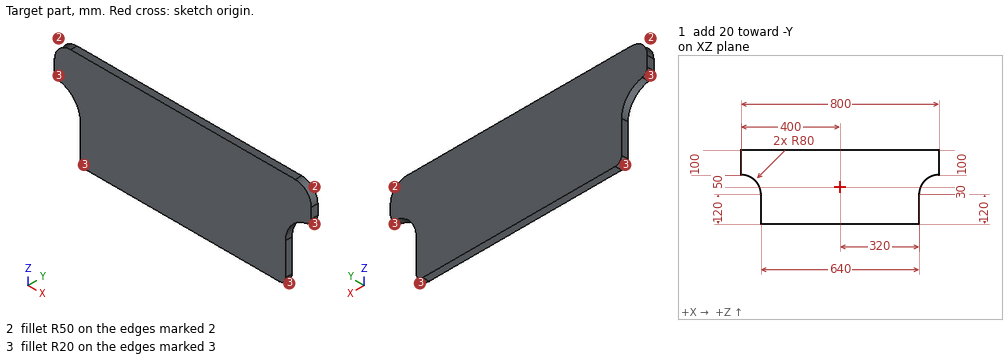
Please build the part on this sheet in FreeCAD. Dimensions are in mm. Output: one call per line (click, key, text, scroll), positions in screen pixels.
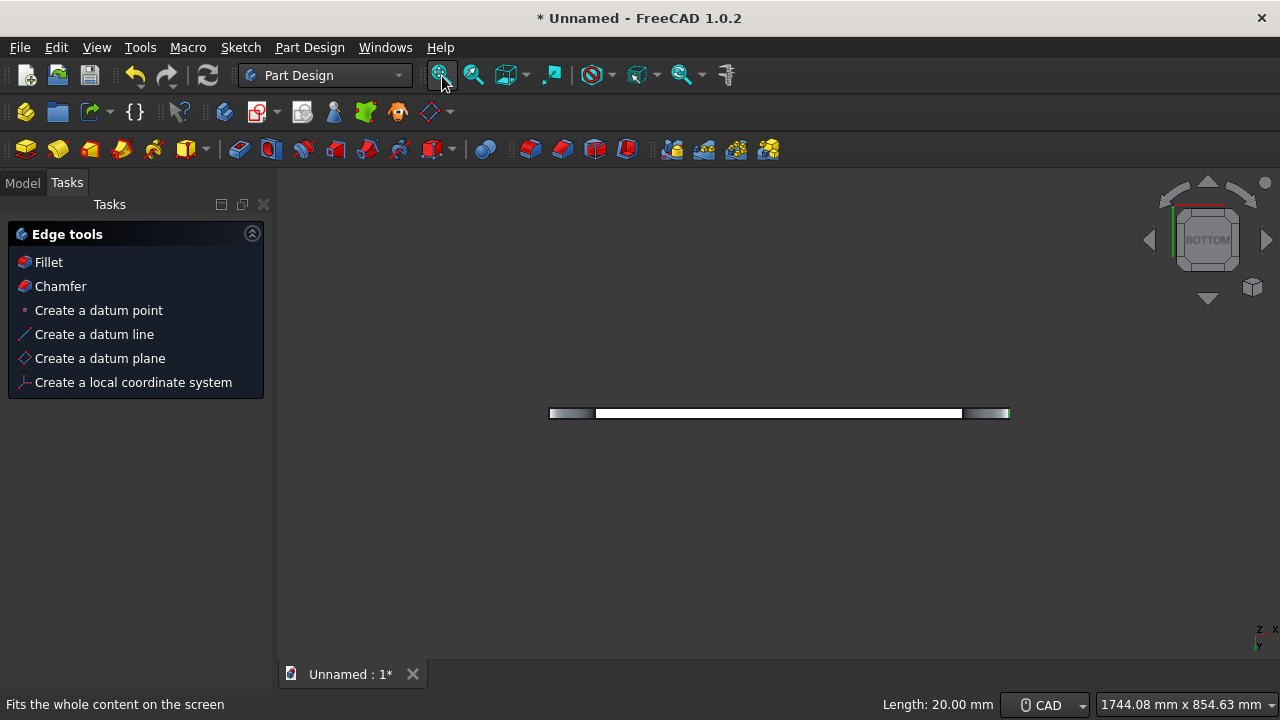
click(595, 414, ctrl)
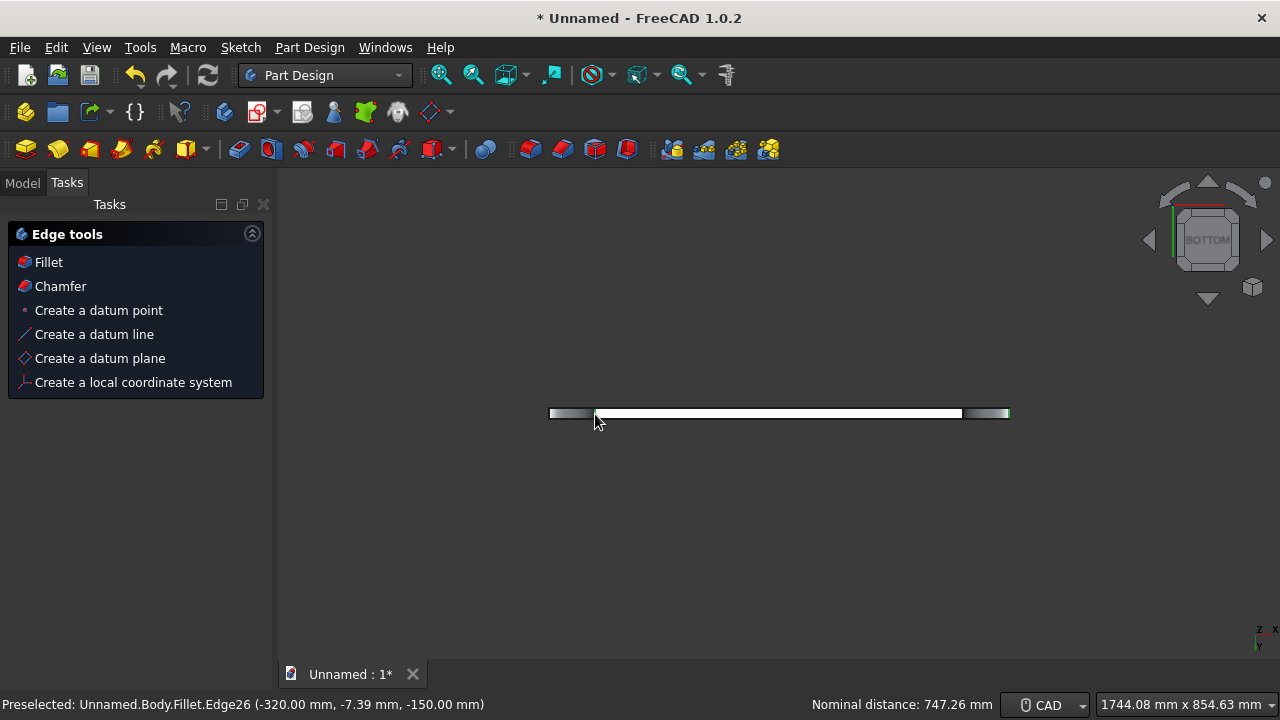
click(963, 414, ctrl)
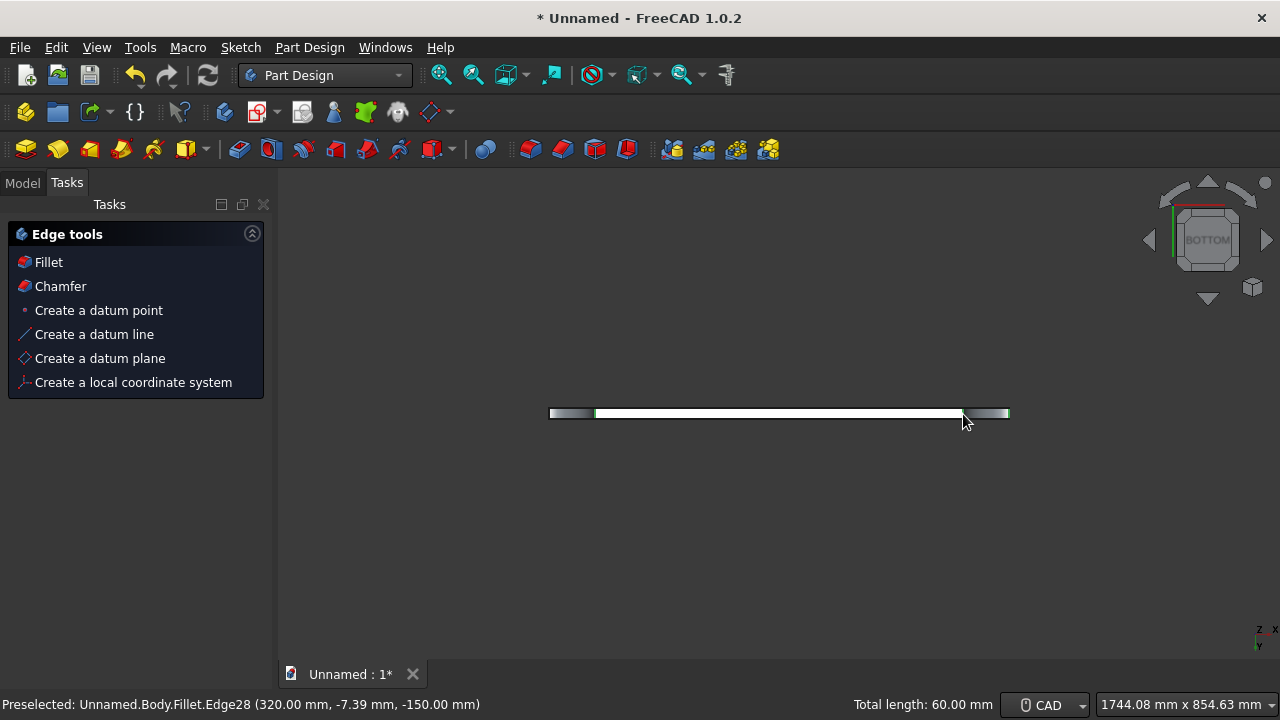
scroll(549, 412, up, 7)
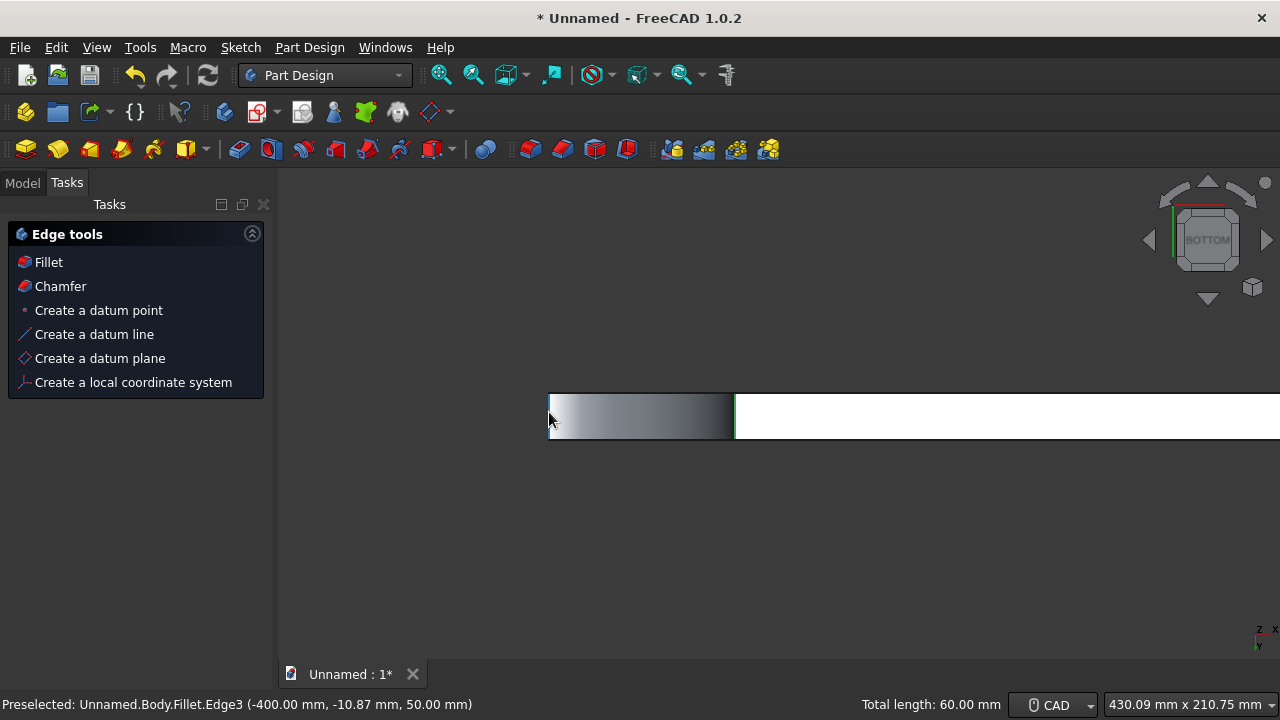
click(442, 76)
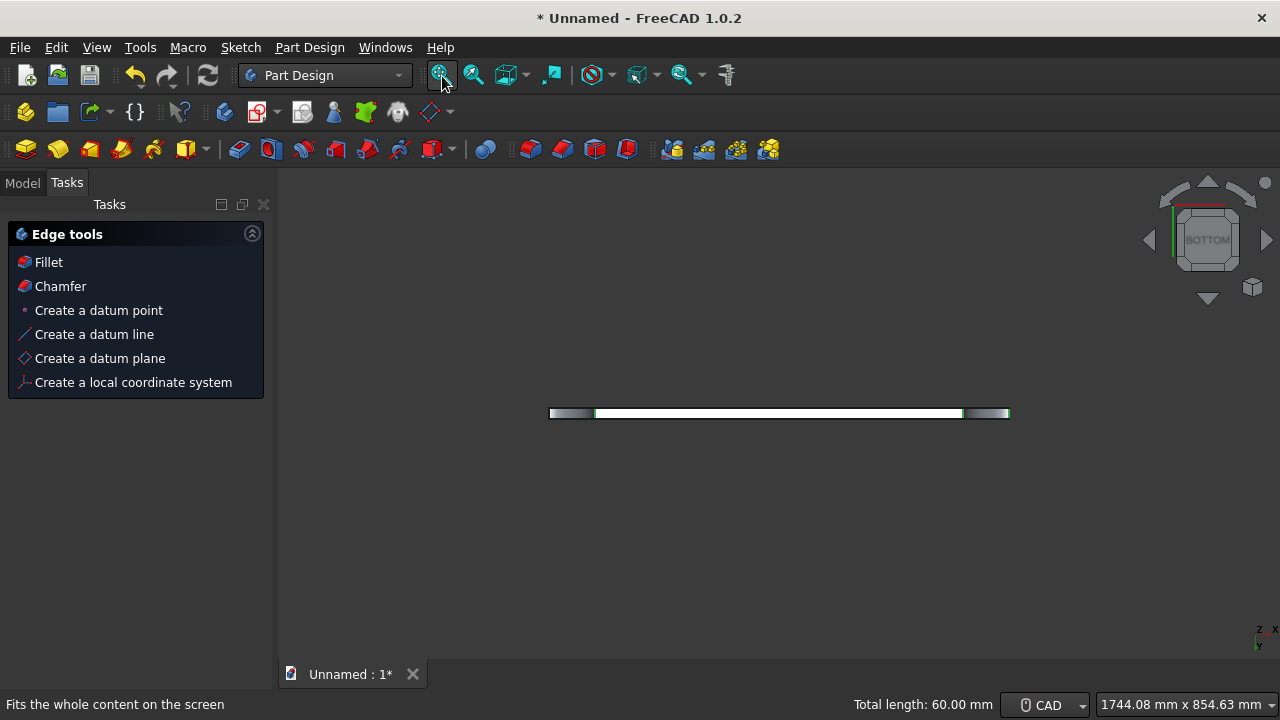
key(4)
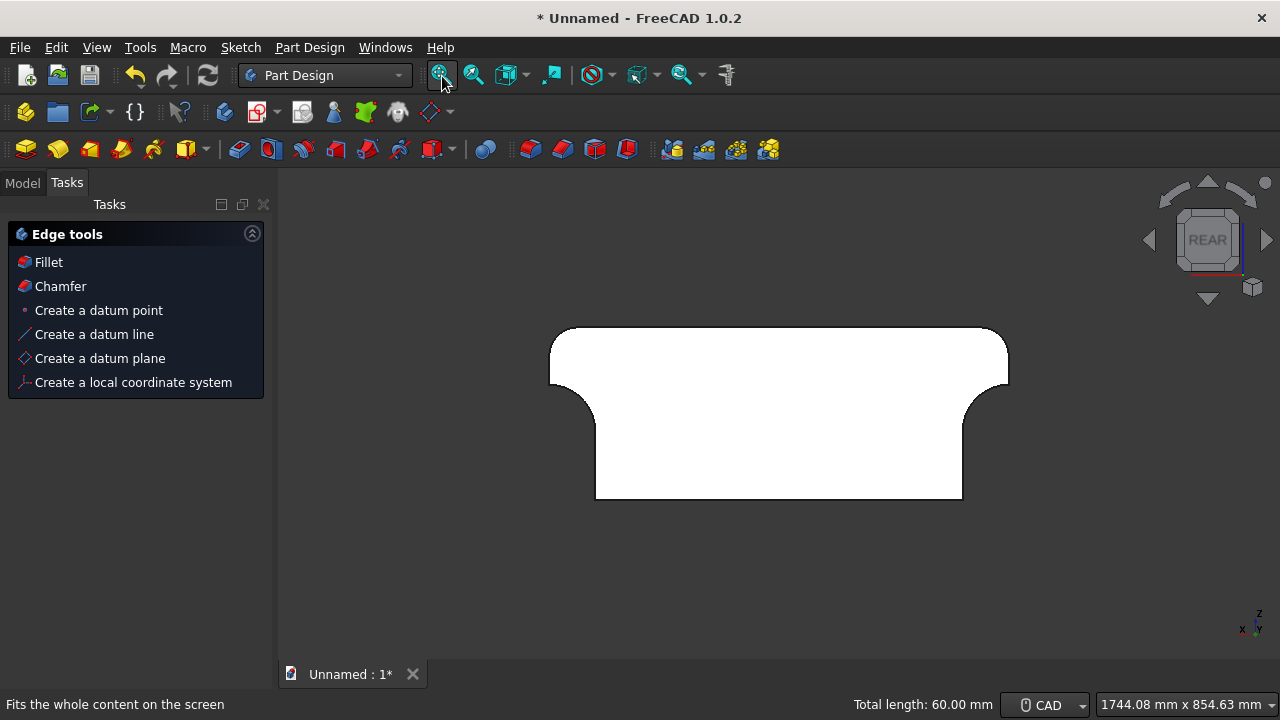
scroll(1009, 384, up, 7)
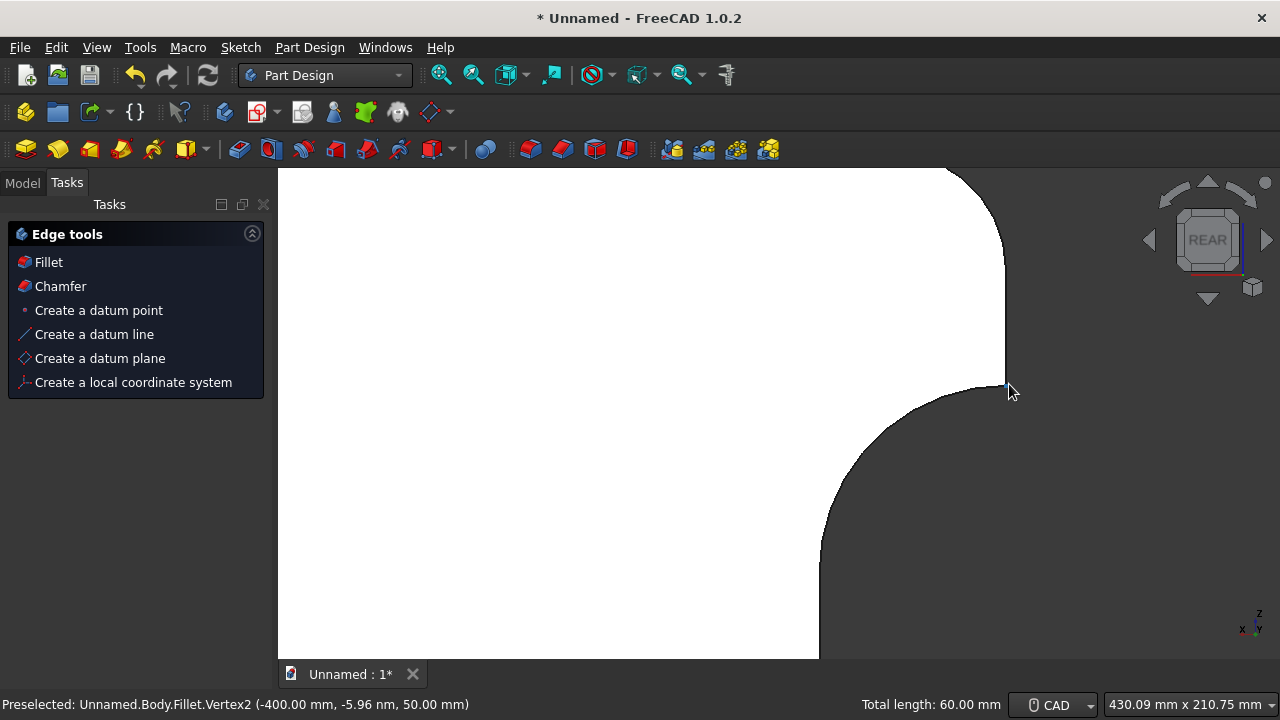
key(v)
key(f)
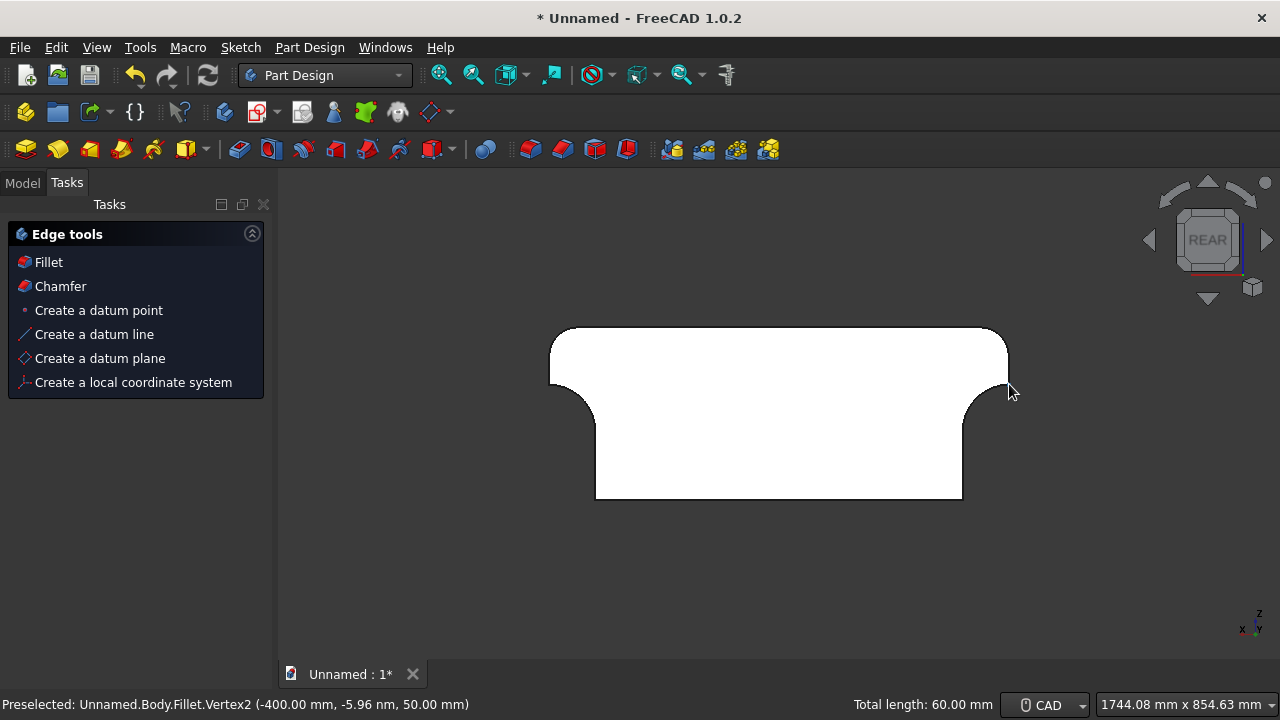
key(6)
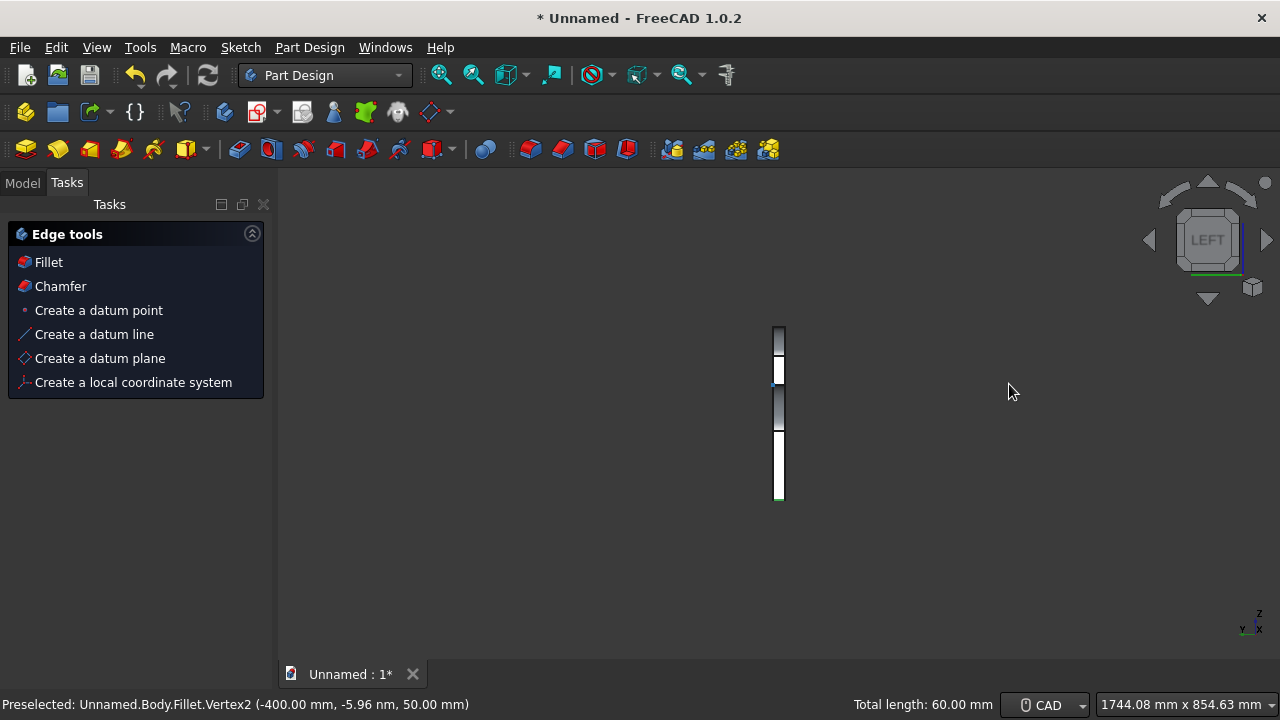
click(442, 76)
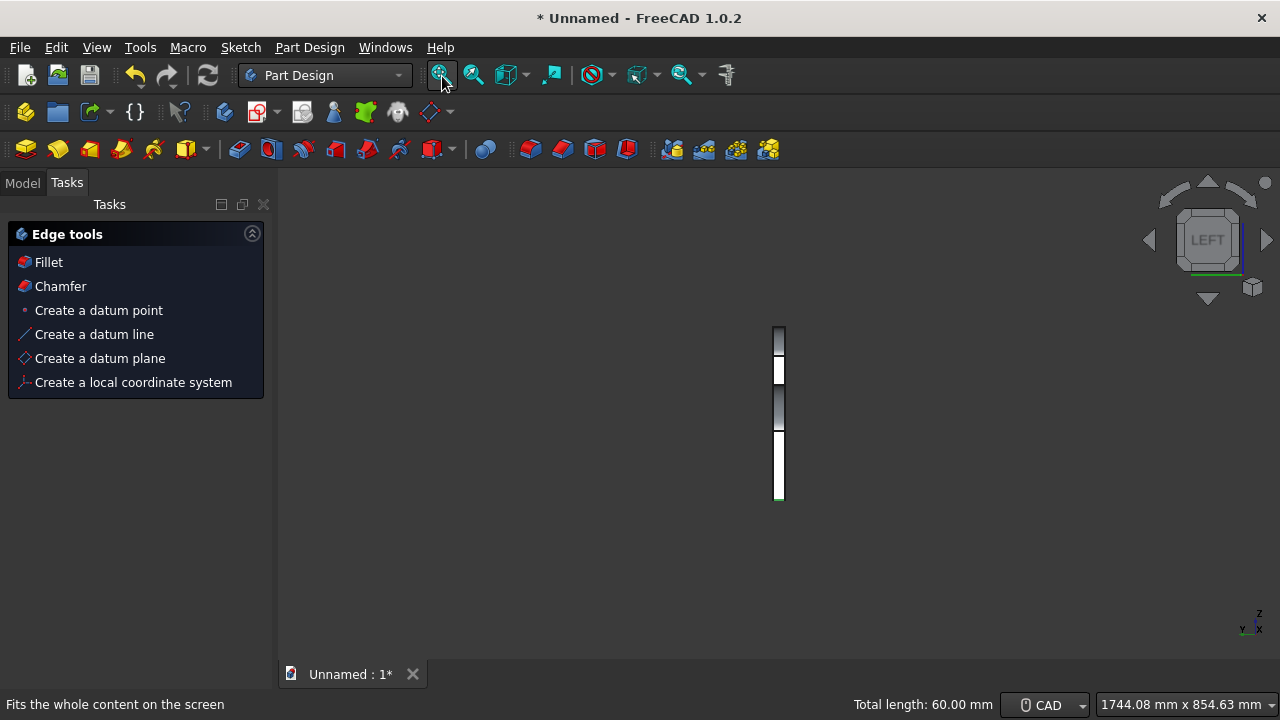
scroll(779, 384, up, 7)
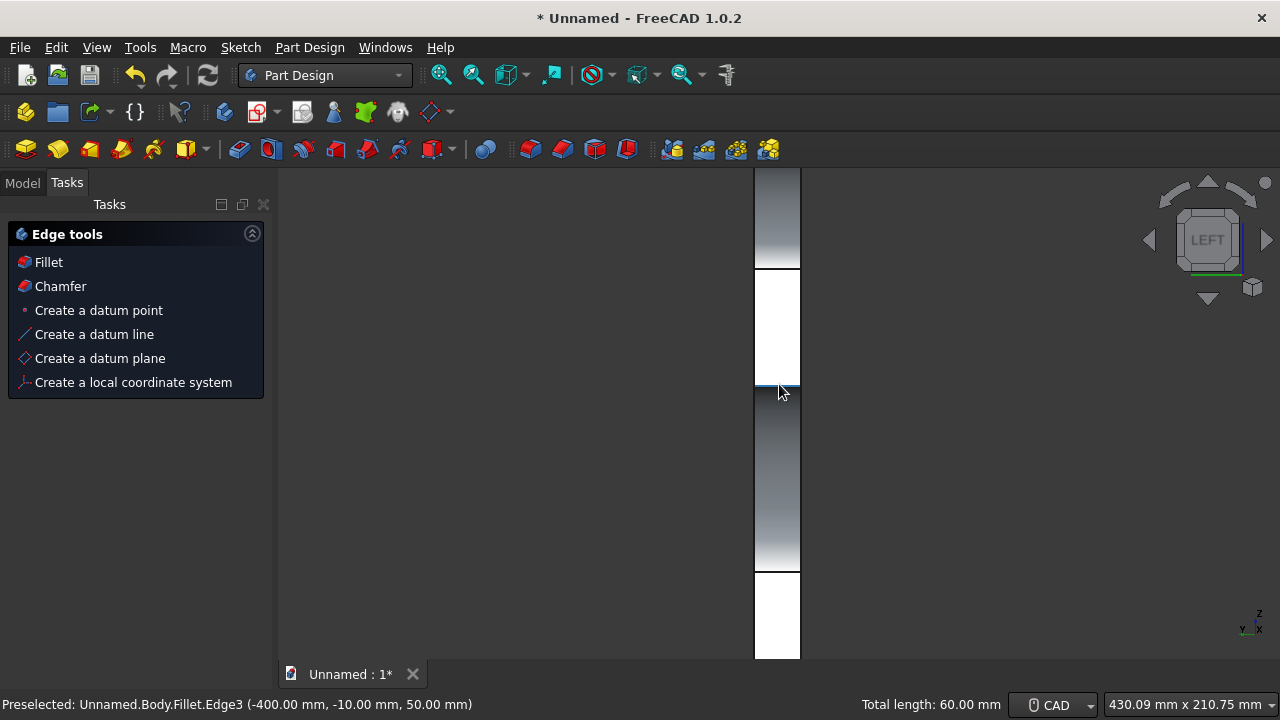
click(777, 385, ctrl)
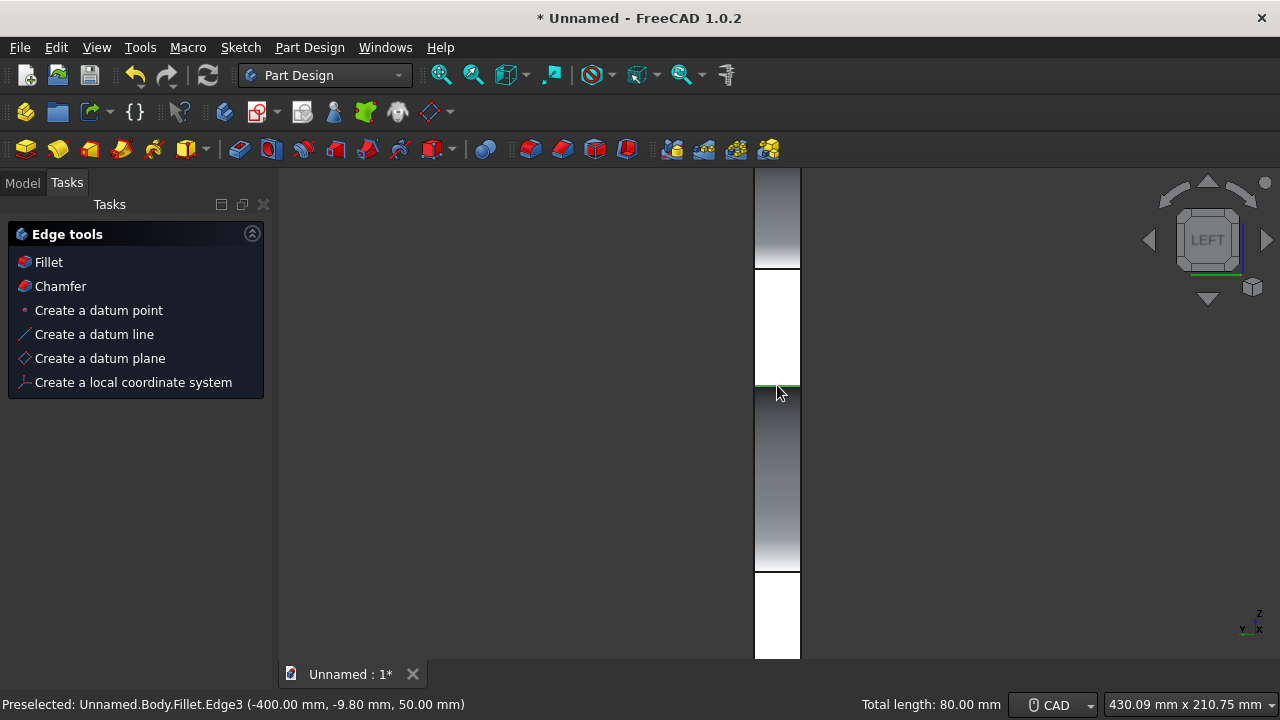
click(532, 150)